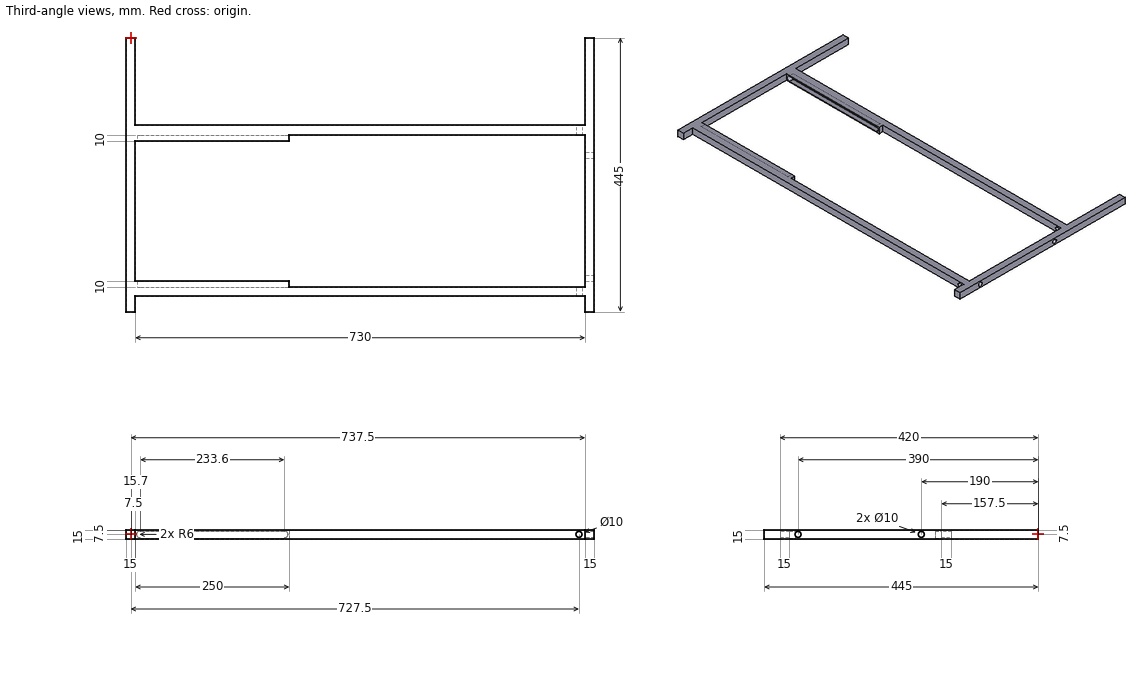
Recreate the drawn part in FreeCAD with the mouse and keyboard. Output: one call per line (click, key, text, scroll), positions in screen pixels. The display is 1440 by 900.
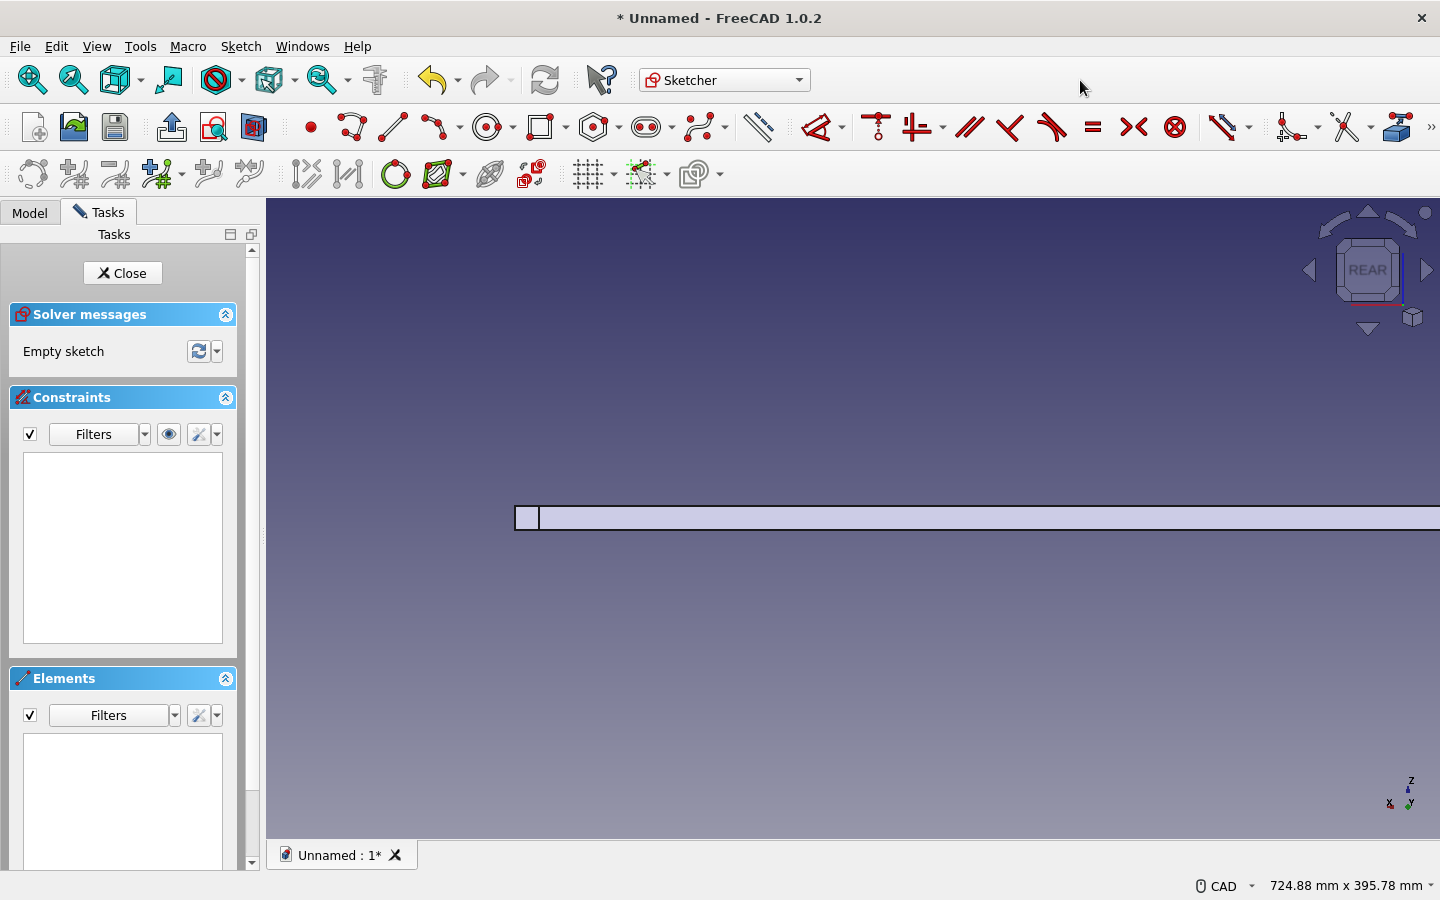
scroll(543, 518, up, 15)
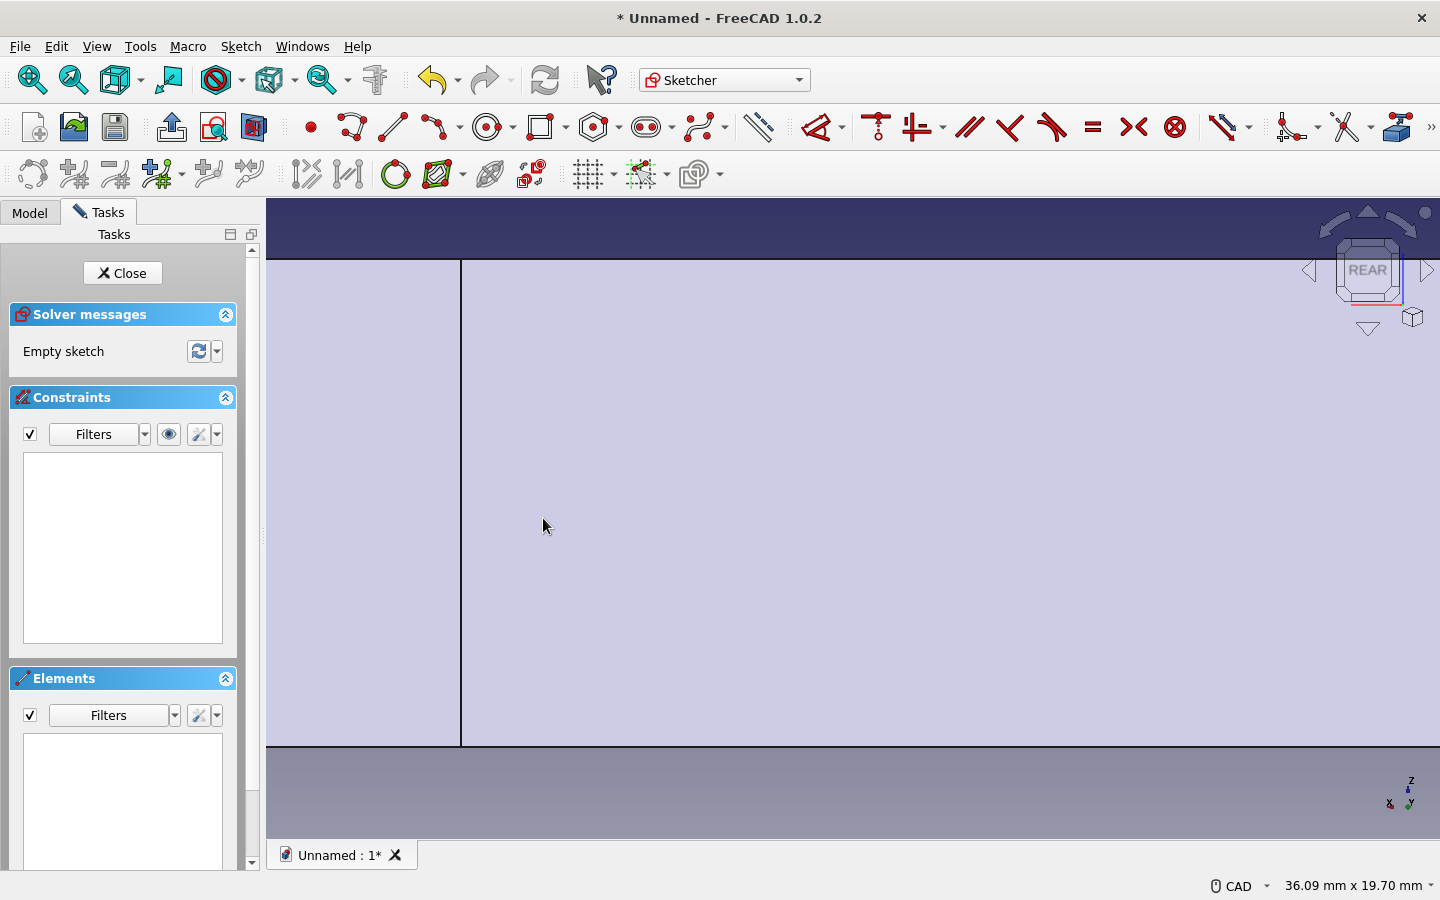
click(486, 128)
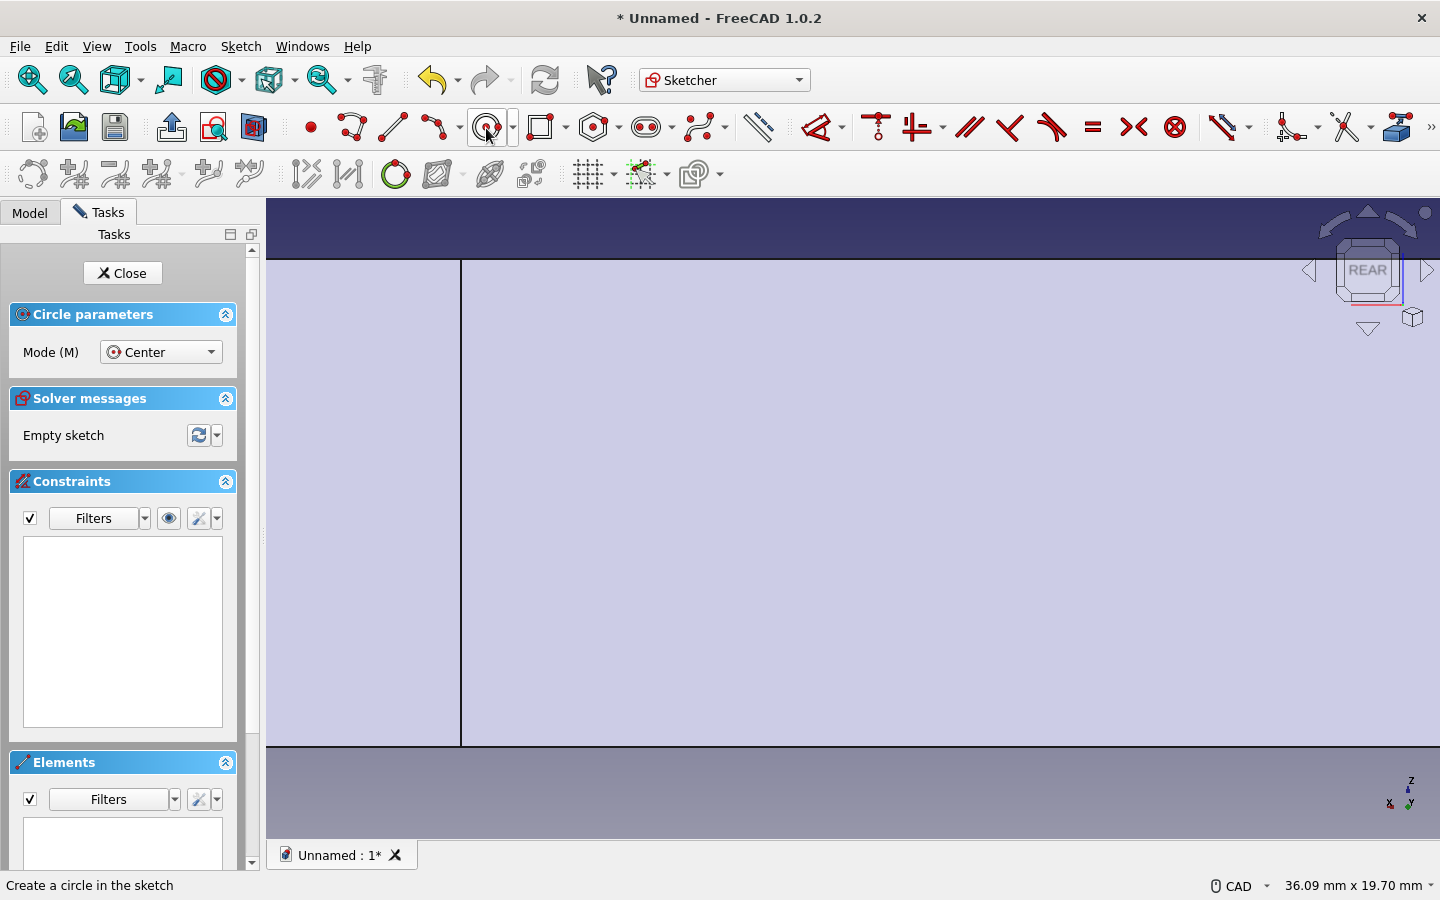
click(786, 503)
click(901, 388)
key(Escape)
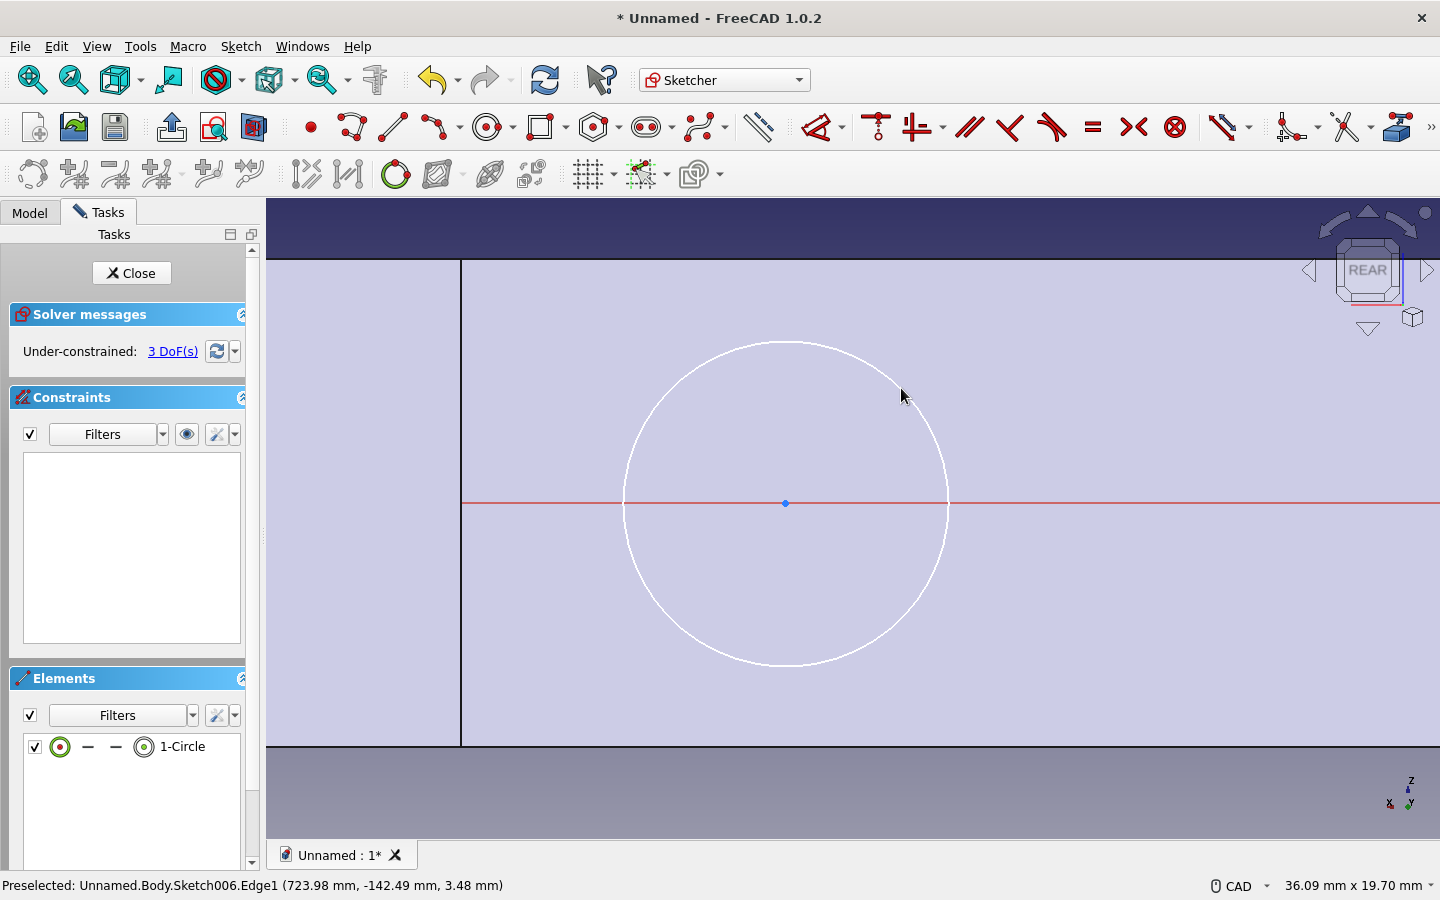
click(786, 504)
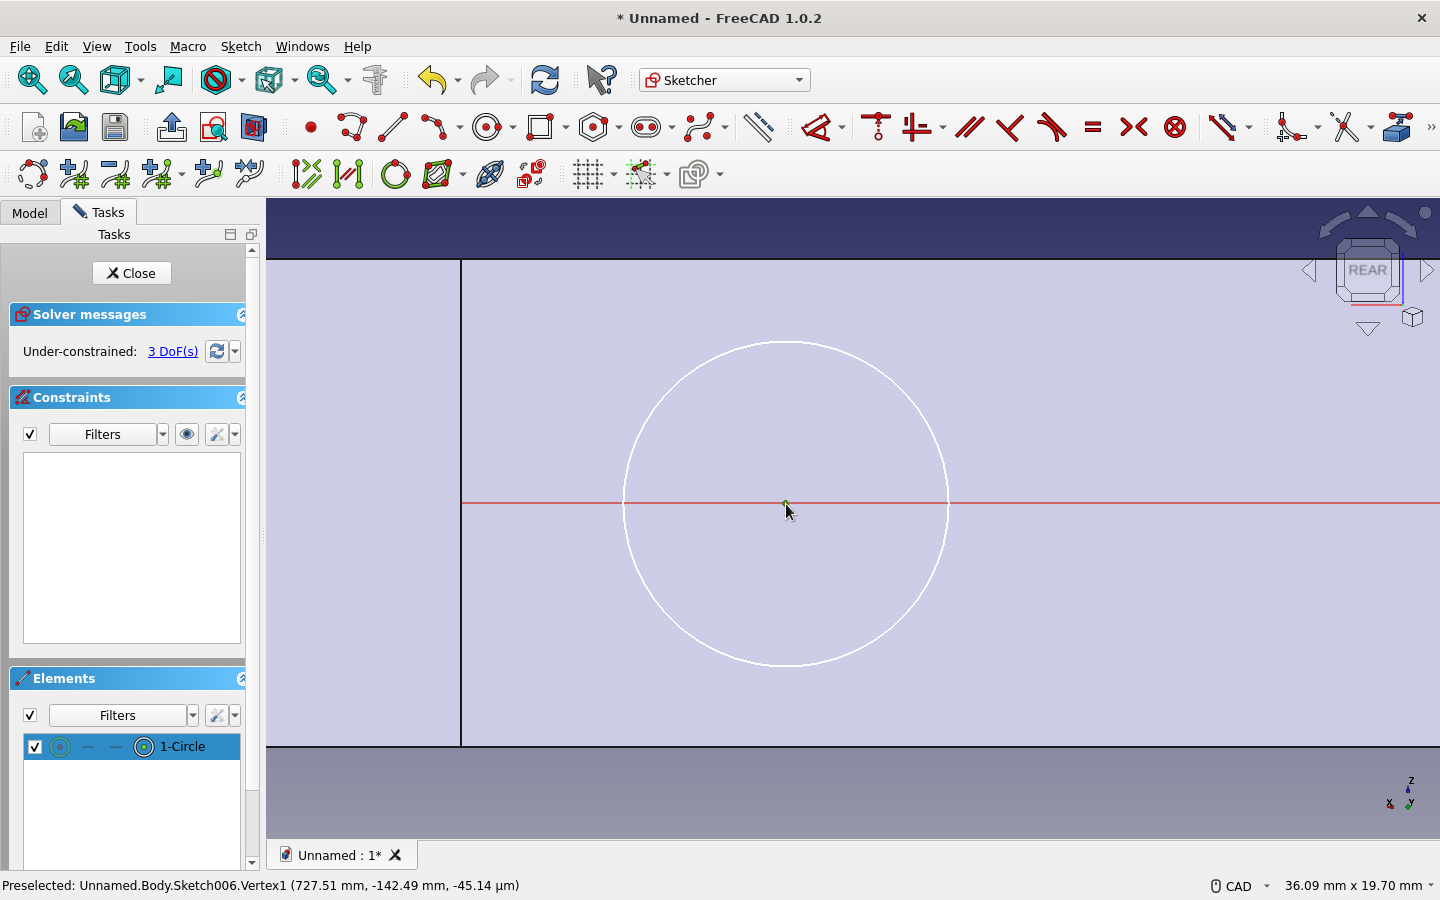
click(364, 503)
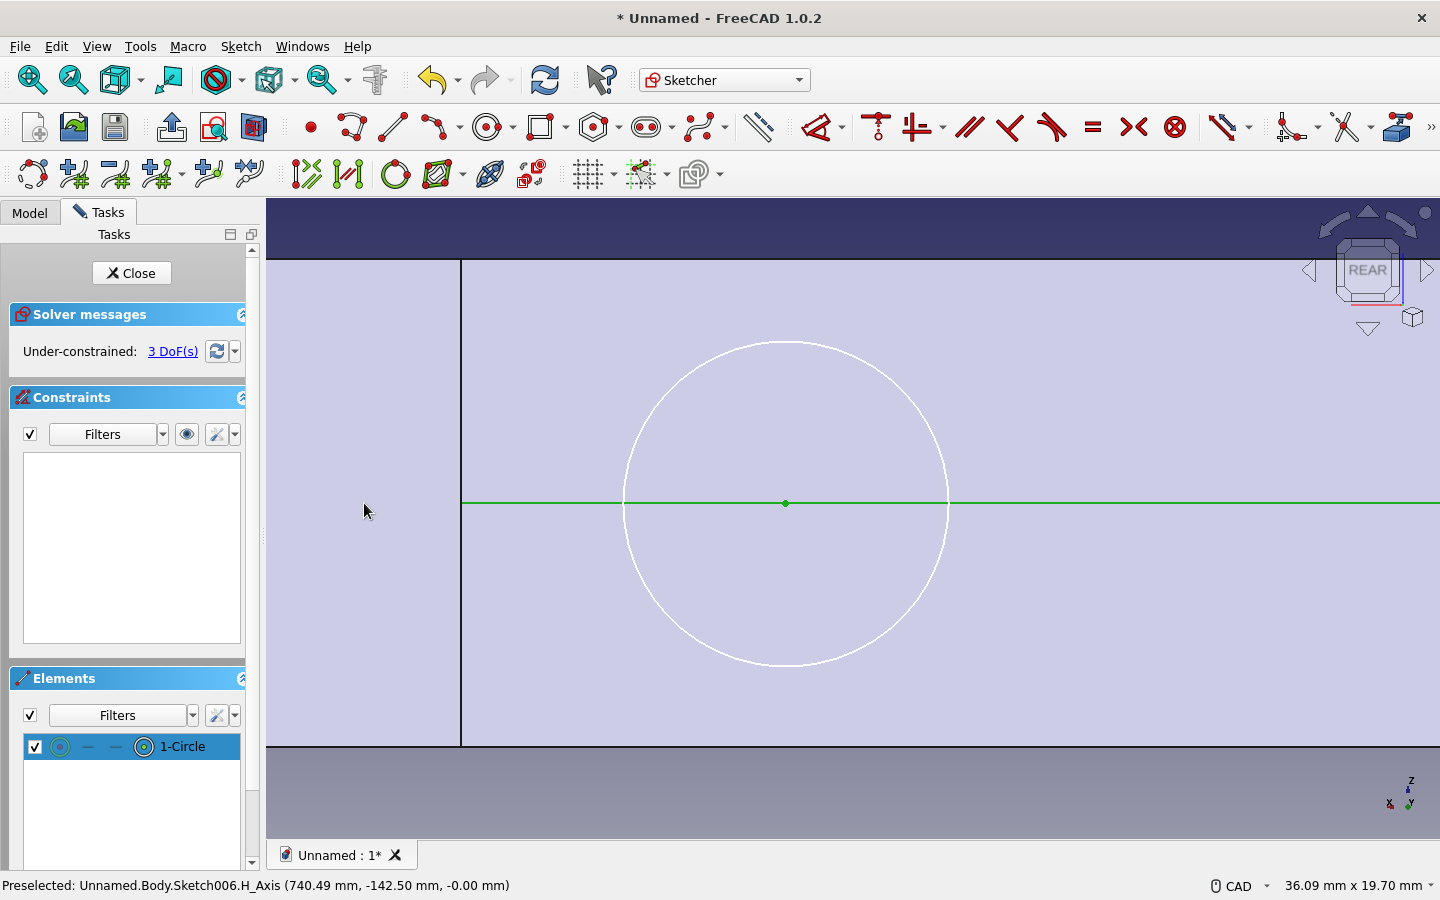
click(876, 128)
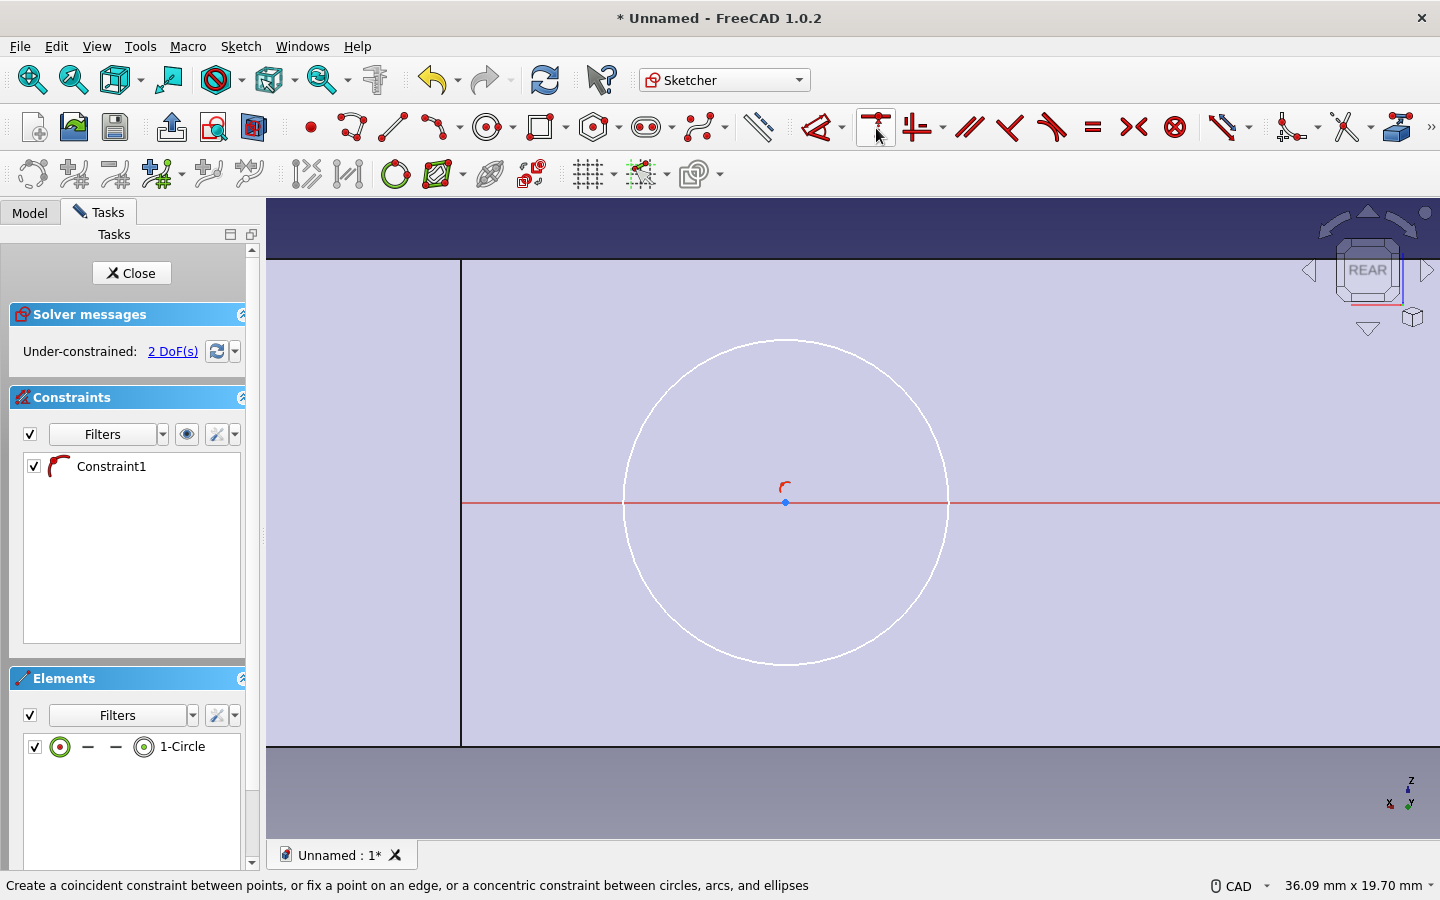
click(816, 128)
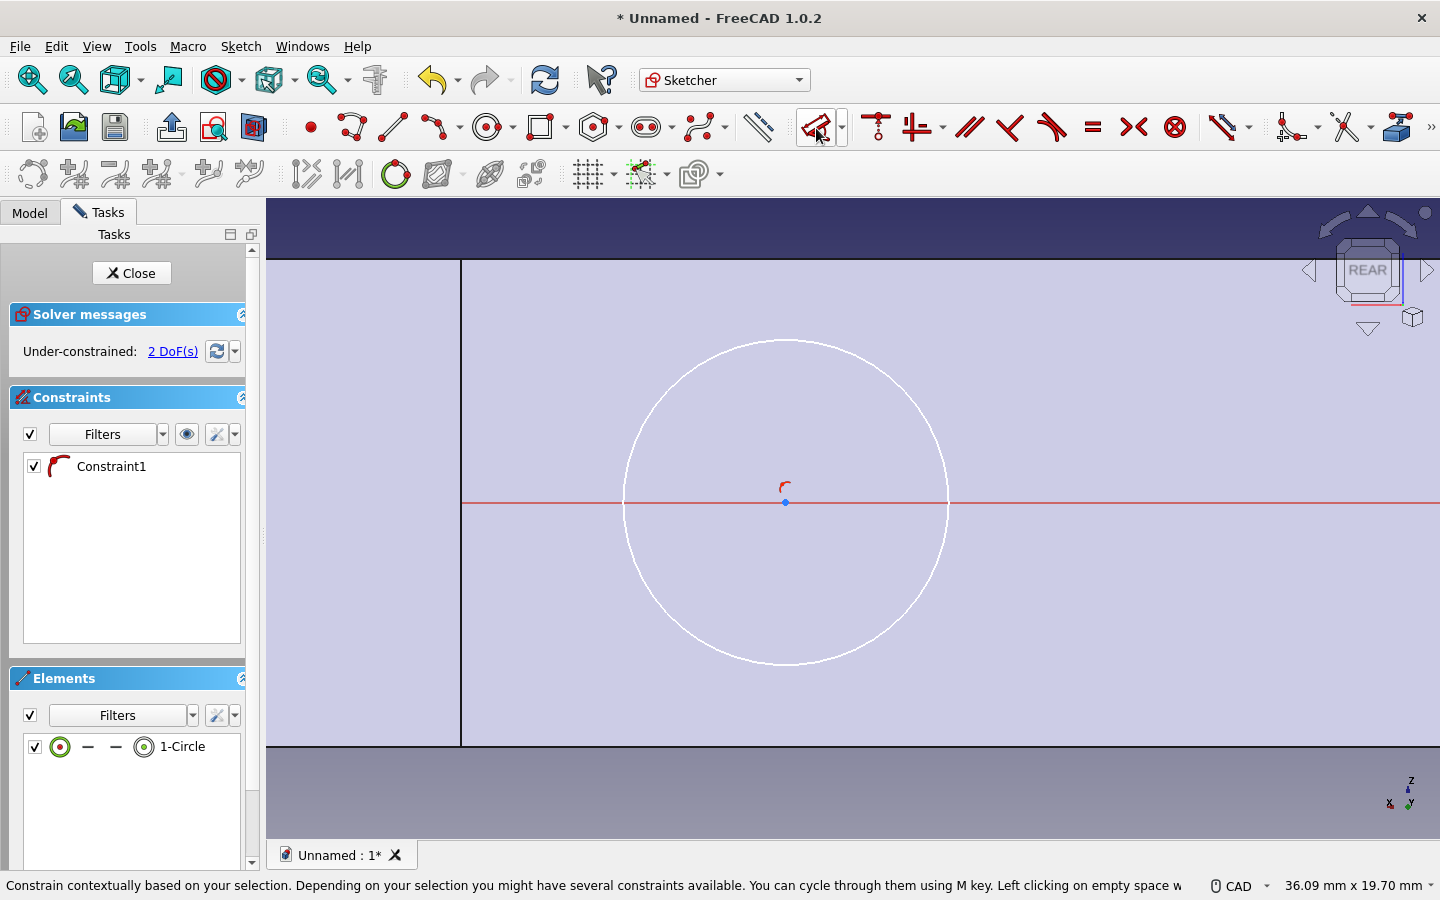
click(901, 387)
click(924, 364)